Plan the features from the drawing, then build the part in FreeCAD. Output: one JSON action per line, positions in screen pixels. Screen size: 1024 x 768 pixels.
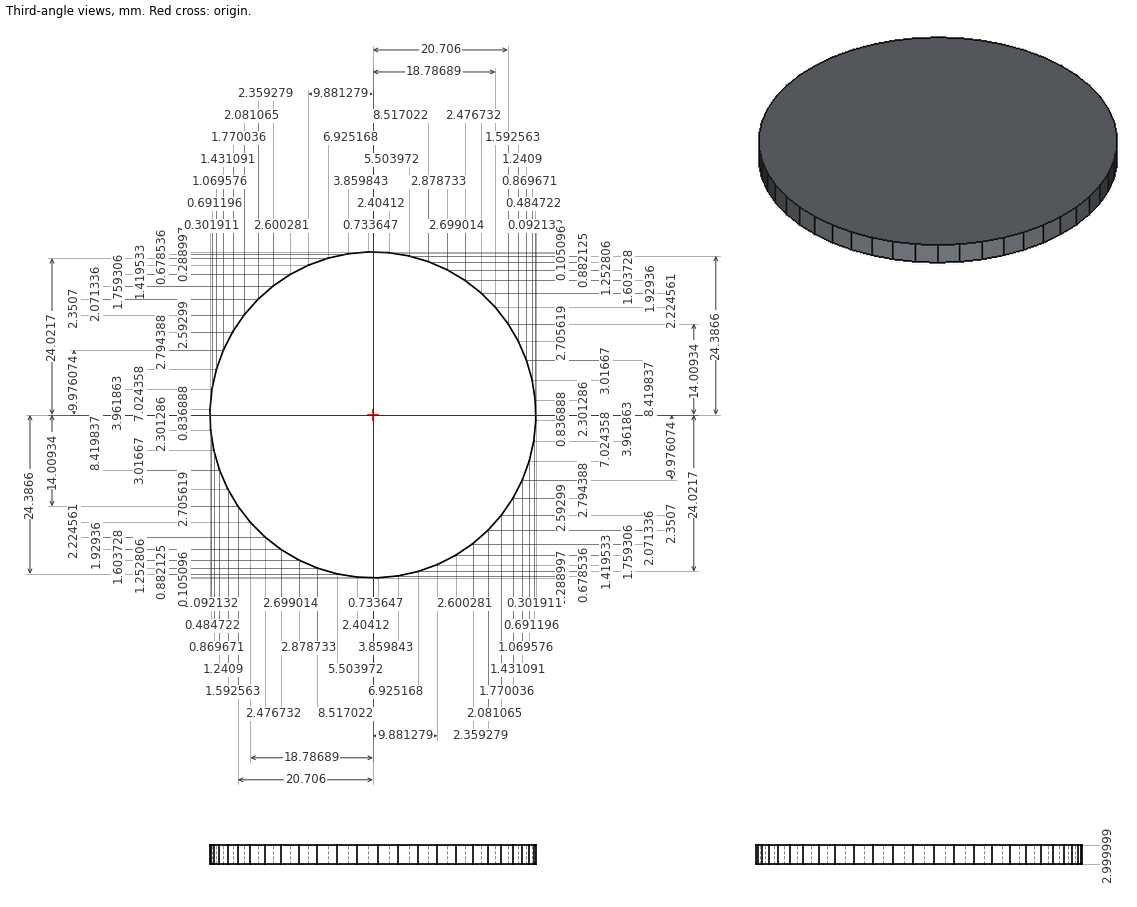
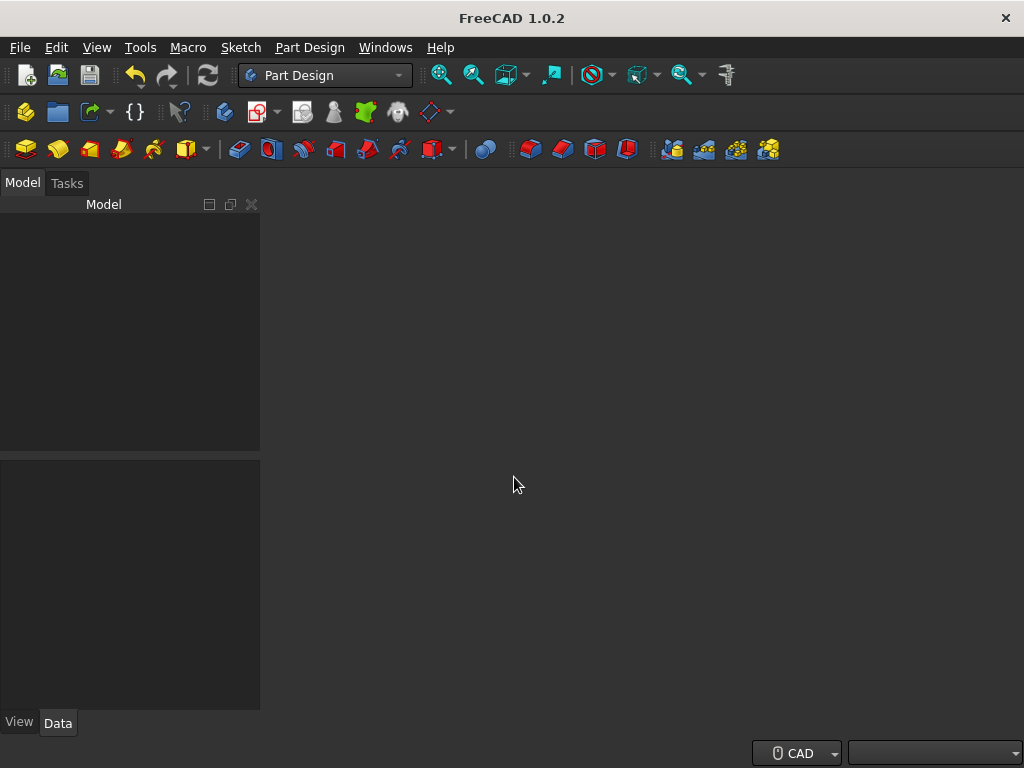
{"action": "left_click", "coordinate": [26, 76]}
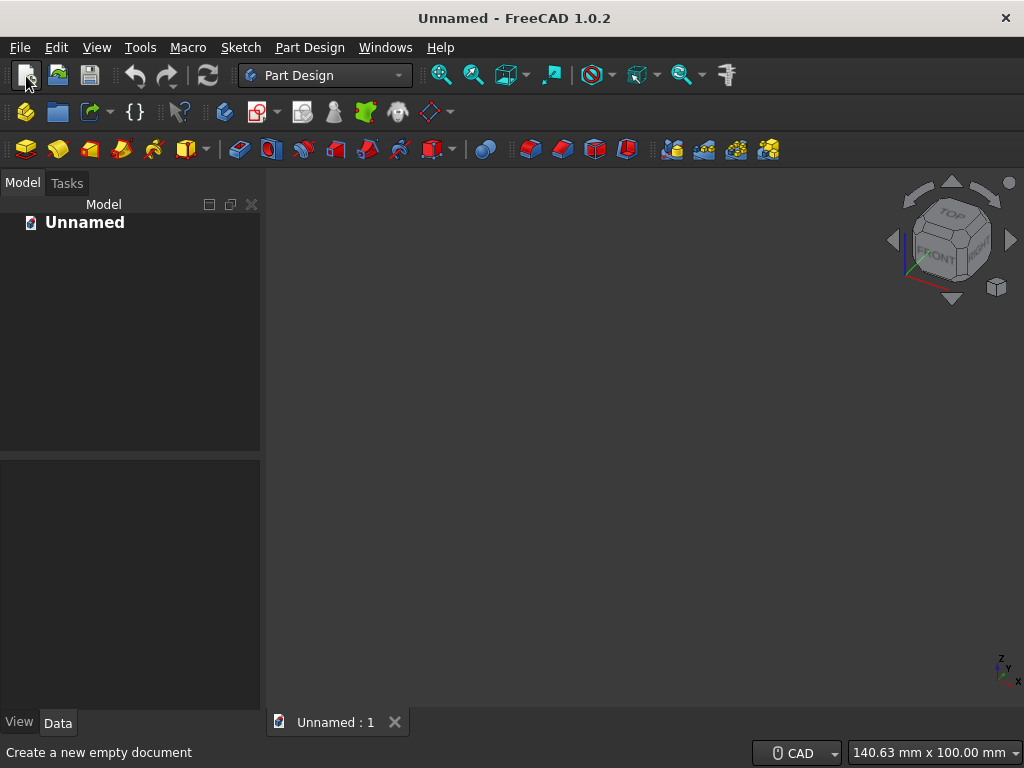
{"action": "left_click", "coordinate": [226, 112]}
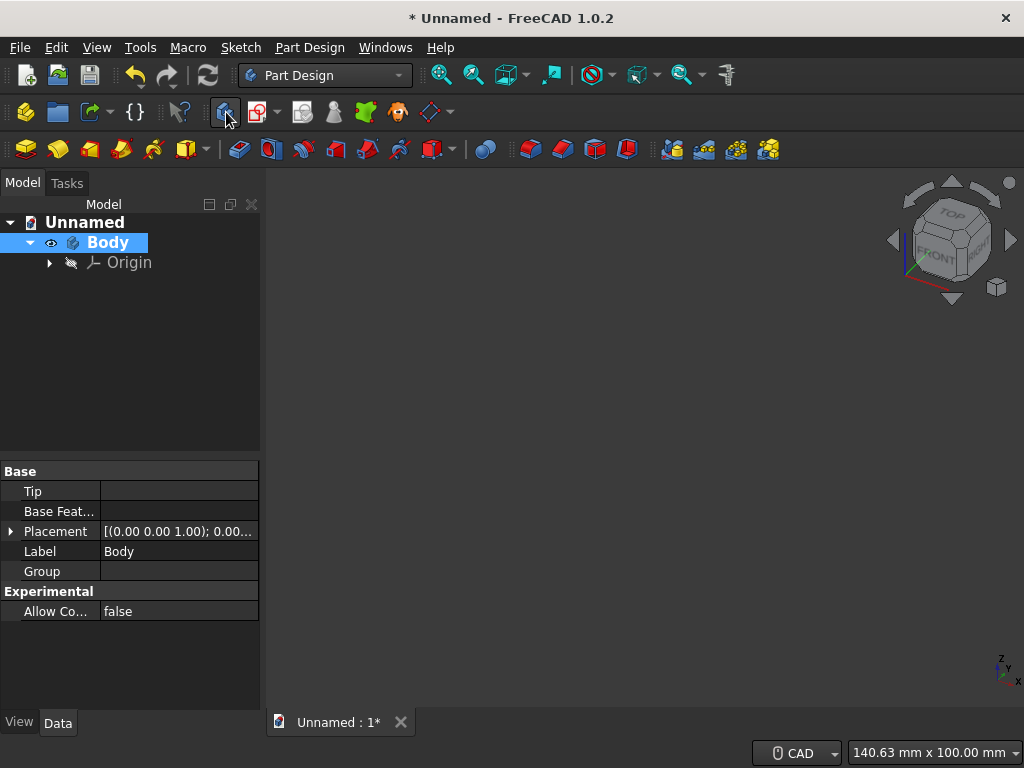
{"action": "left_click", "coordinate": [50, 263]}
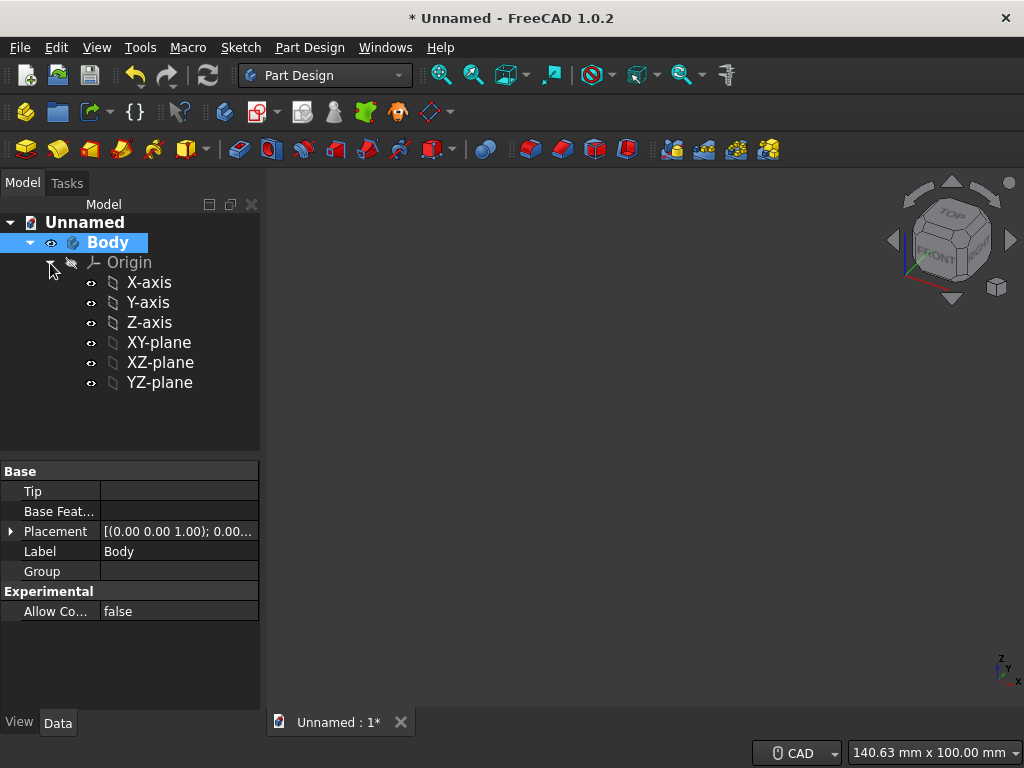
{"action": "left_click", "coordinate": [136, 343]}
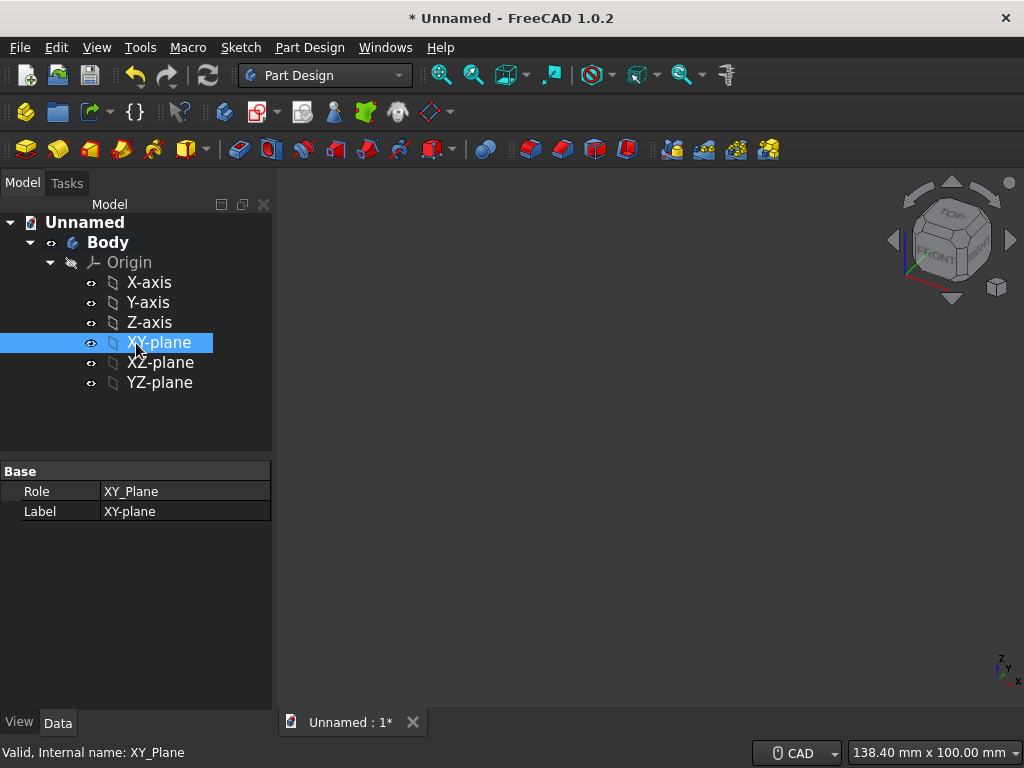
{"action": "left_click", "coordinate": [430, 112]}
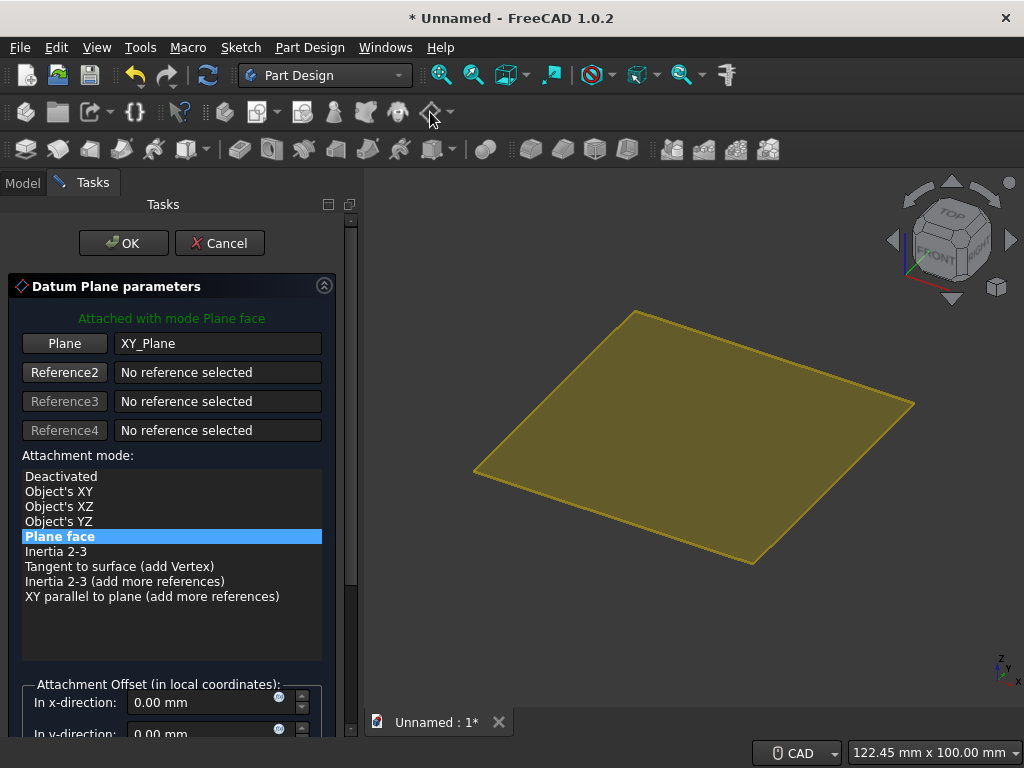
{"action": "scroll", "coordinate": [351, 475], "scroll_direction": "down", "scroll_amount": 2}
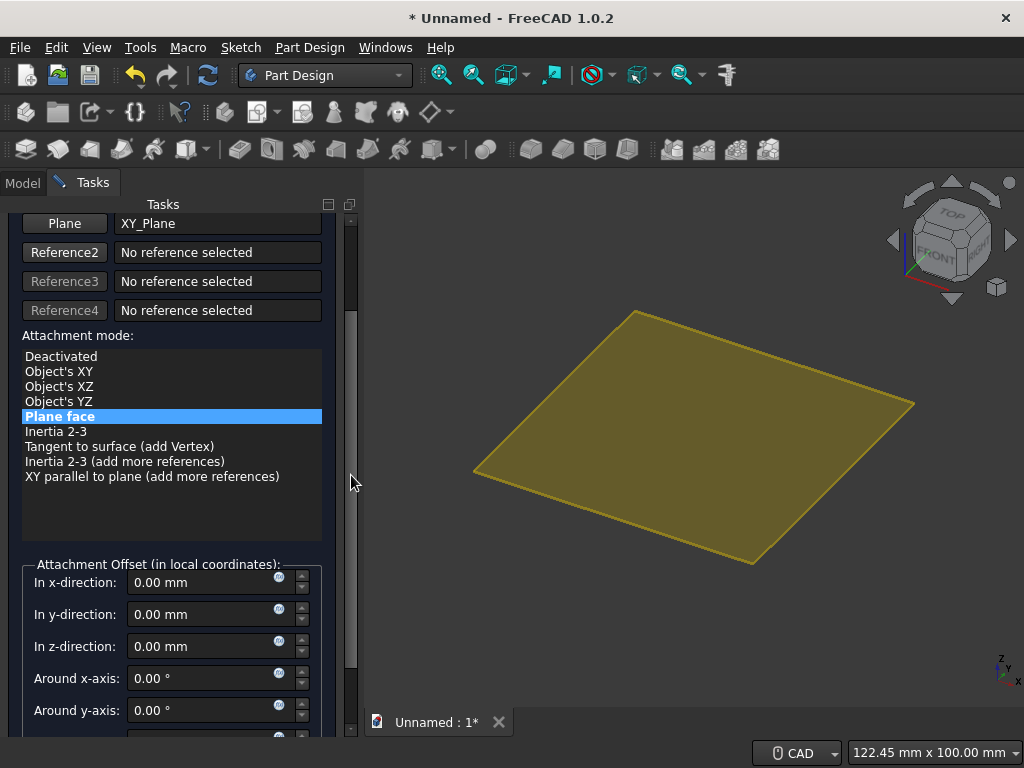
{"action": "triple_click", "coordinate": [210, 646]}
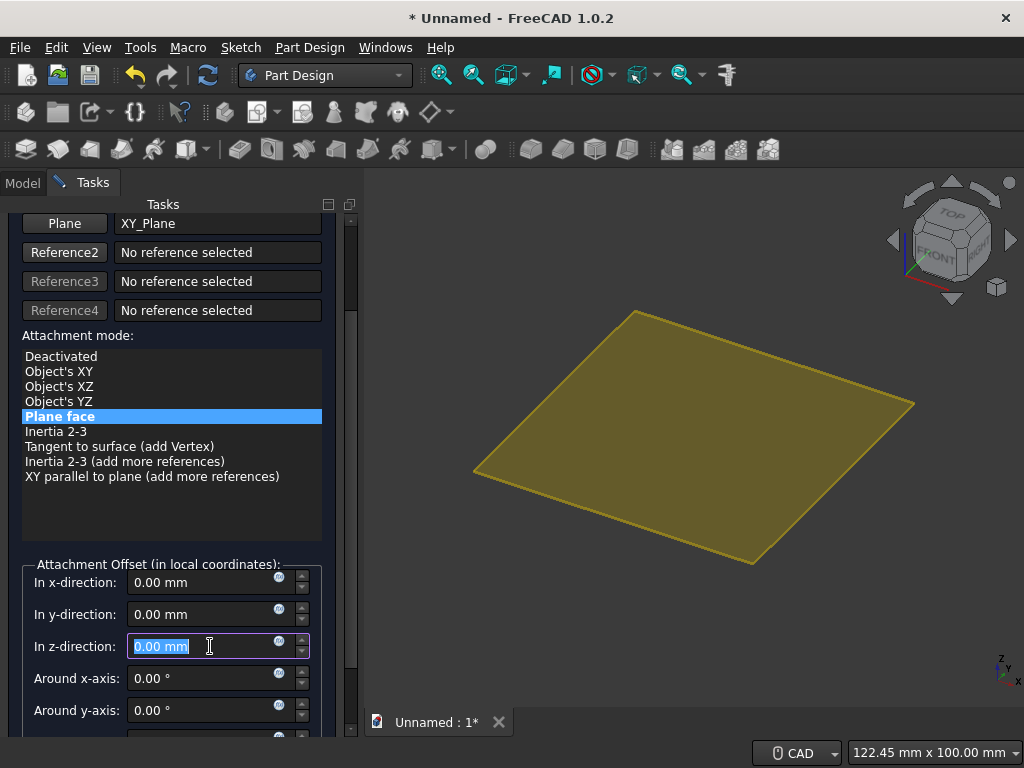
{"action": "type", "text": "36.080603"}
{"action": "key", "text": "Tab"}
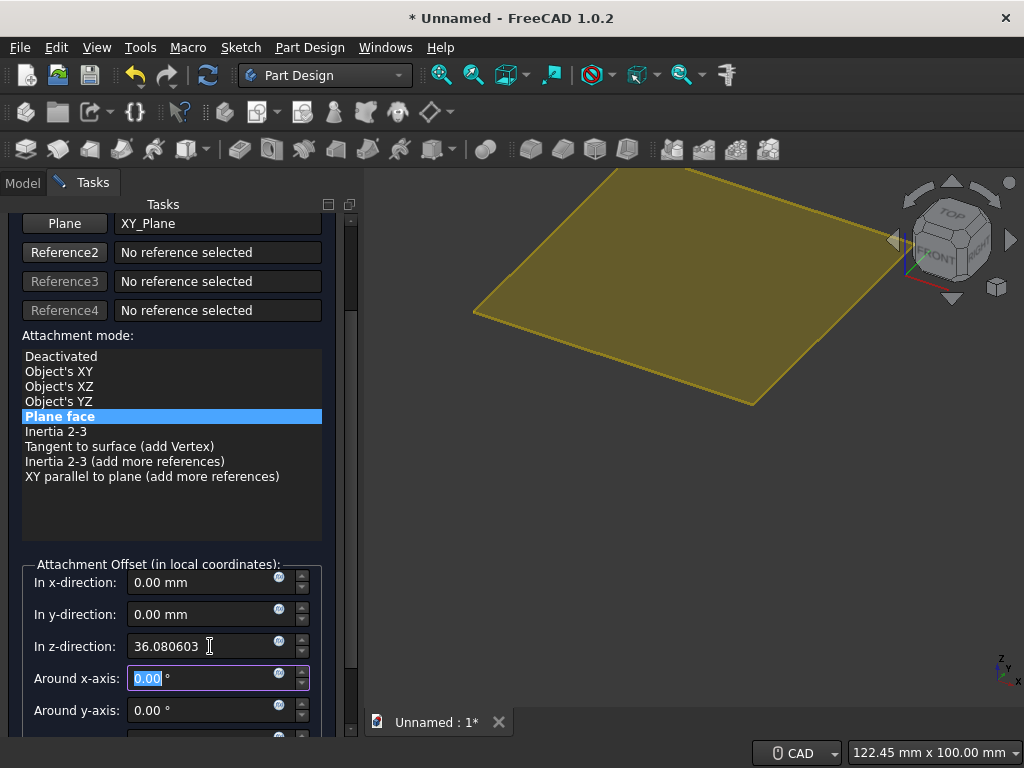
{"action": "scroll", "coordinate": [351, 475], "scroll_direction": "up", "scroll_amount": 3}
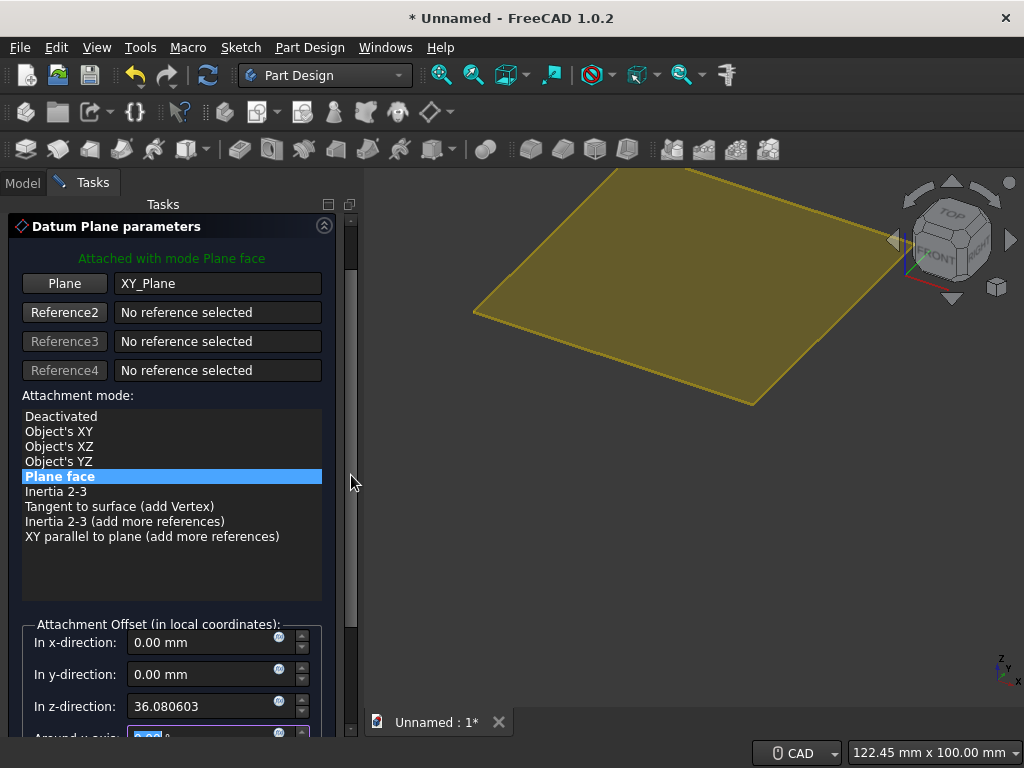
{"action": "left_click", "coordinate": [124, 243]}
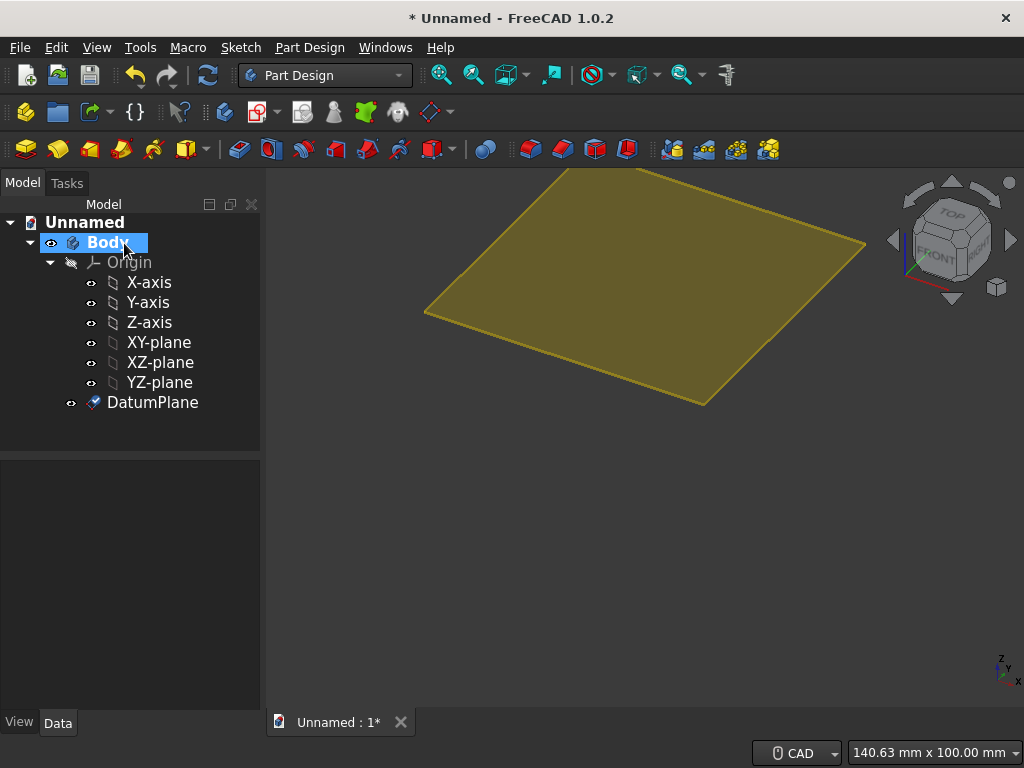
{"action": "left_click", "coordinate": [116, 403]}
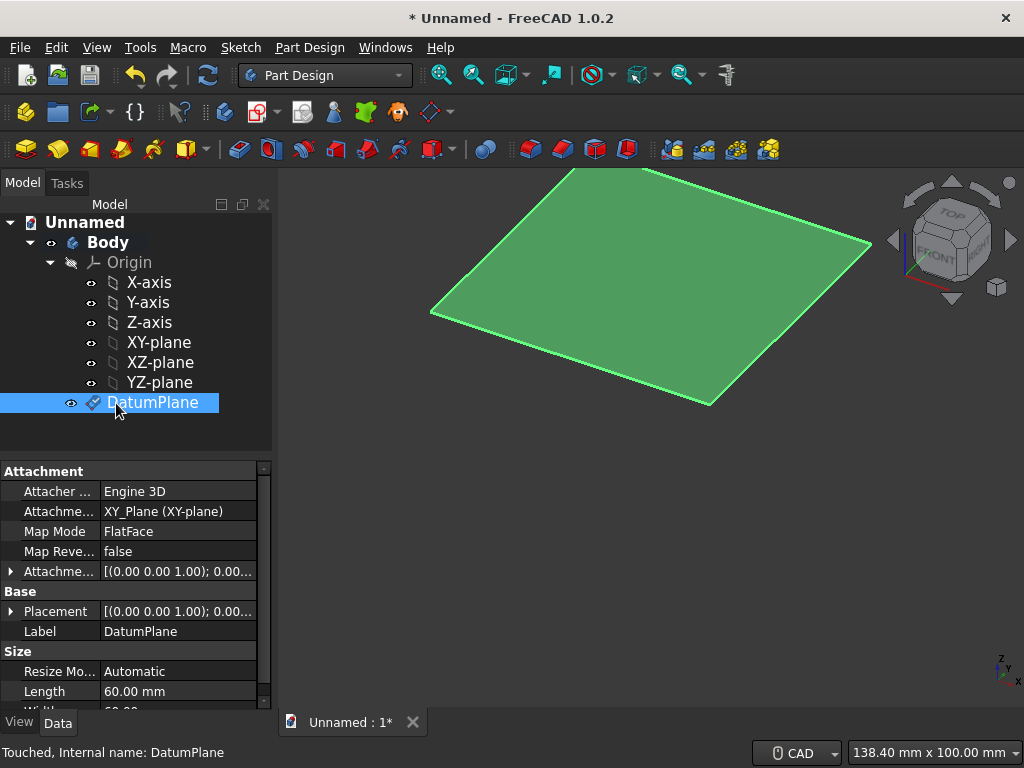
{"action": "left_click", "coordinate": [258, 112]}